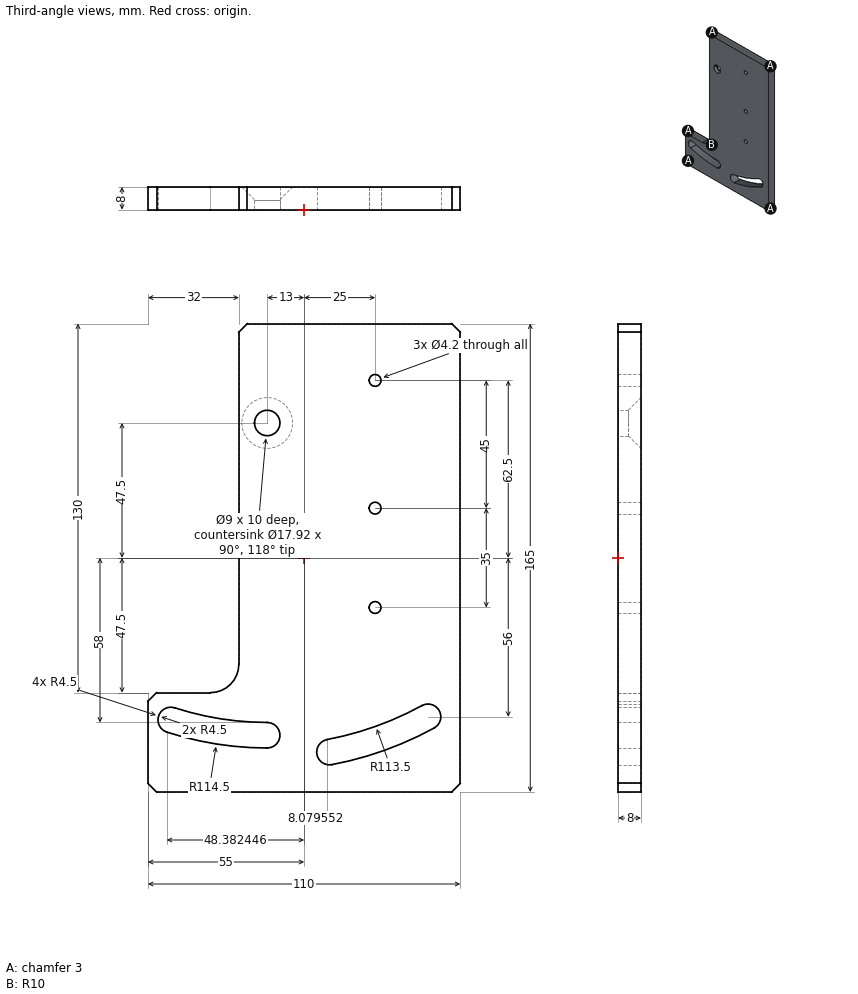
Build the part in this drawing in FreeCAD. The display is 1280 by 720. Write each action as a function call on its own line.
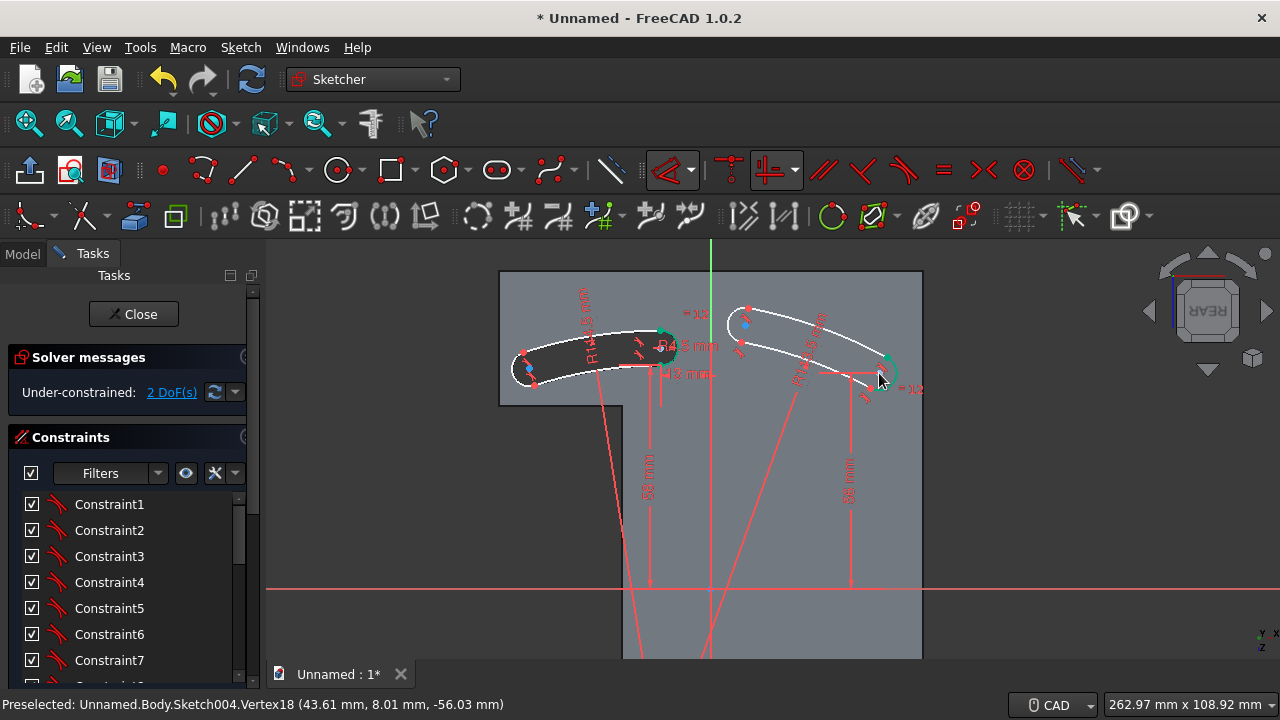
scroll(742, 342, up, 2)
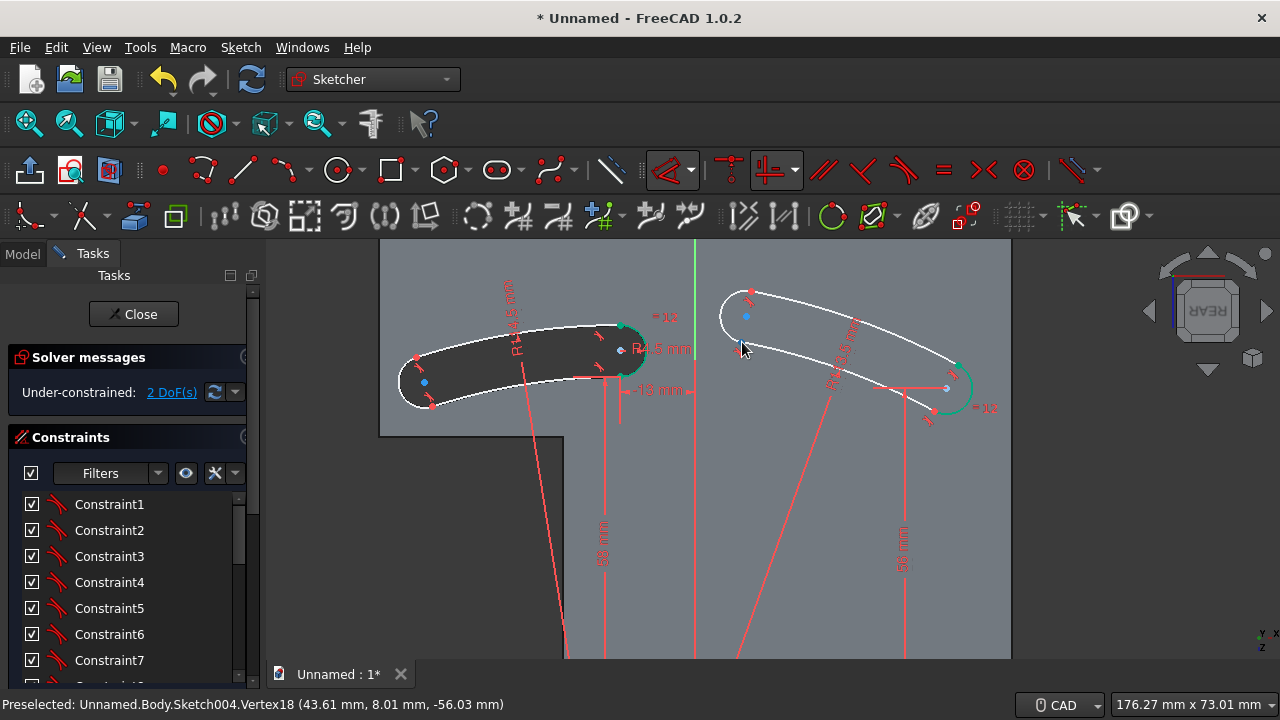
click(741, 342)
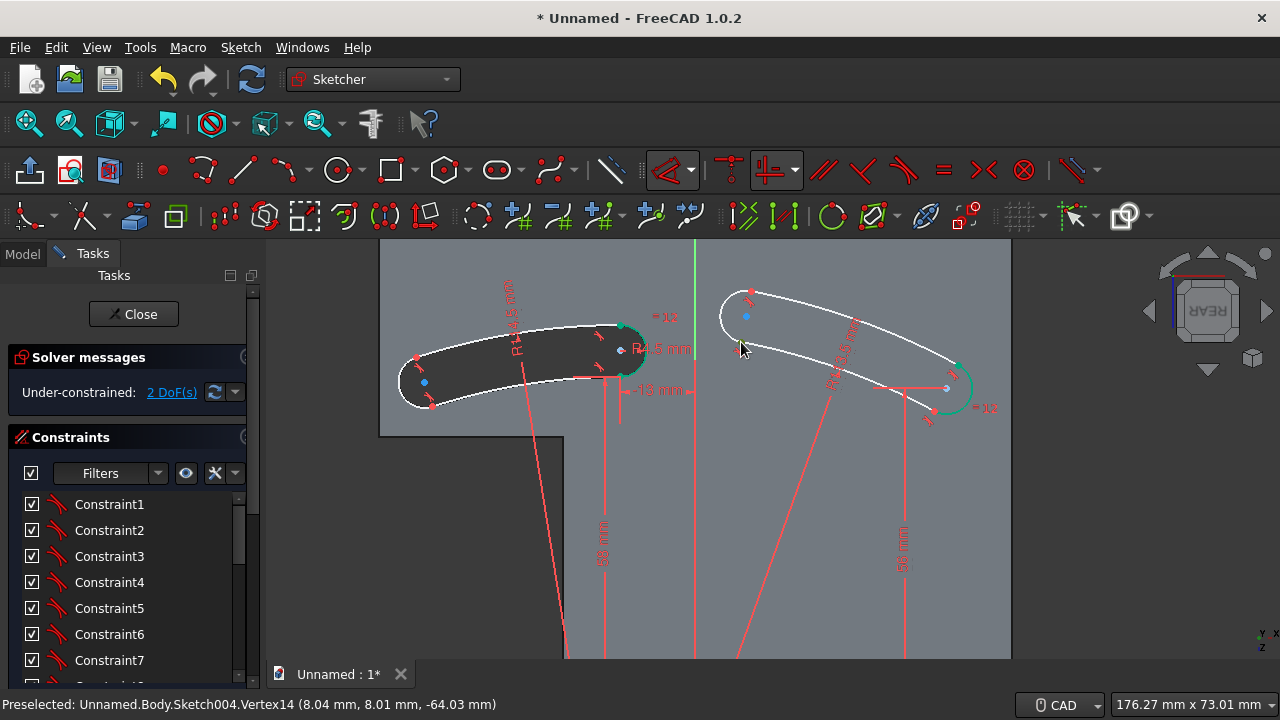
click(694, 170)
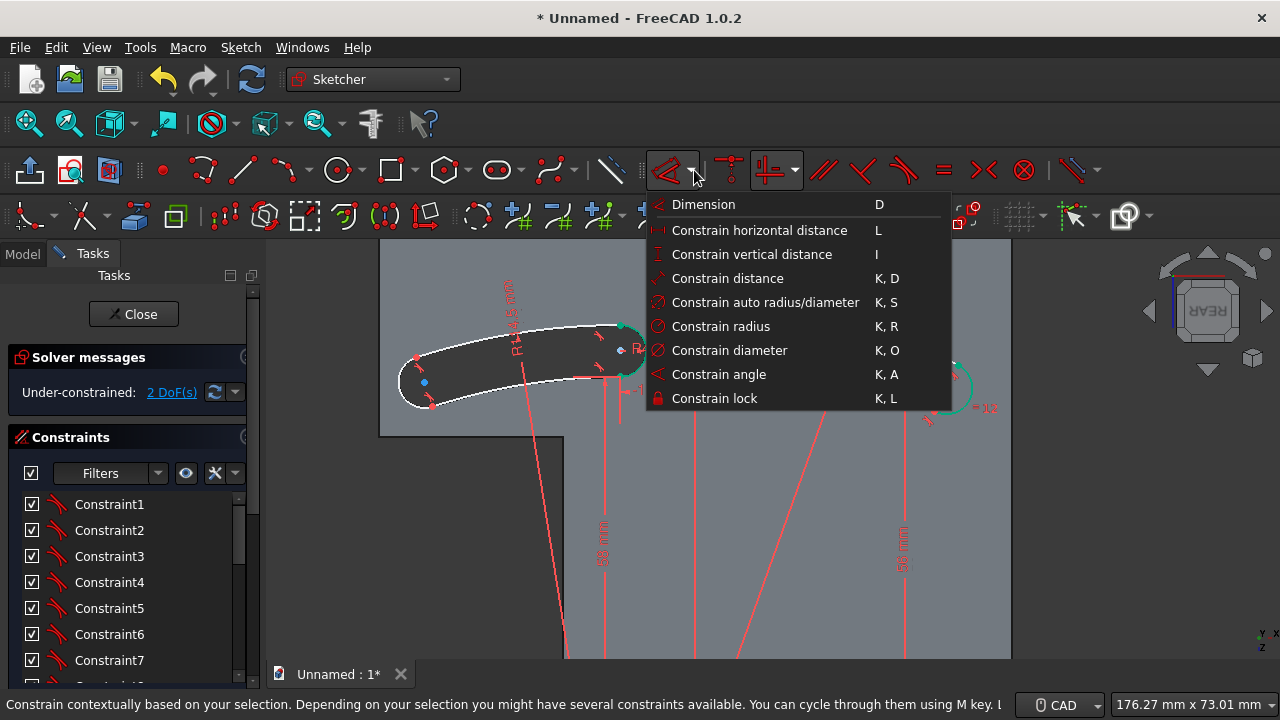
click(799, 230)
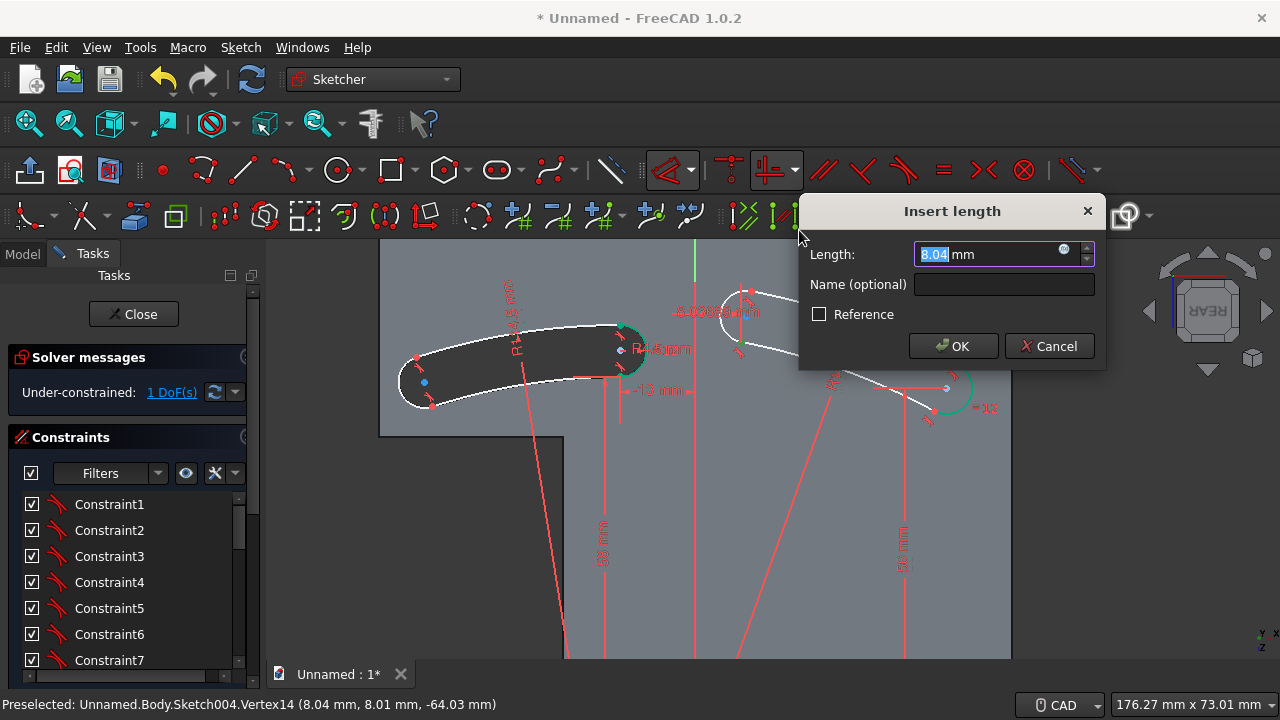
text(8.079552)
key(Return)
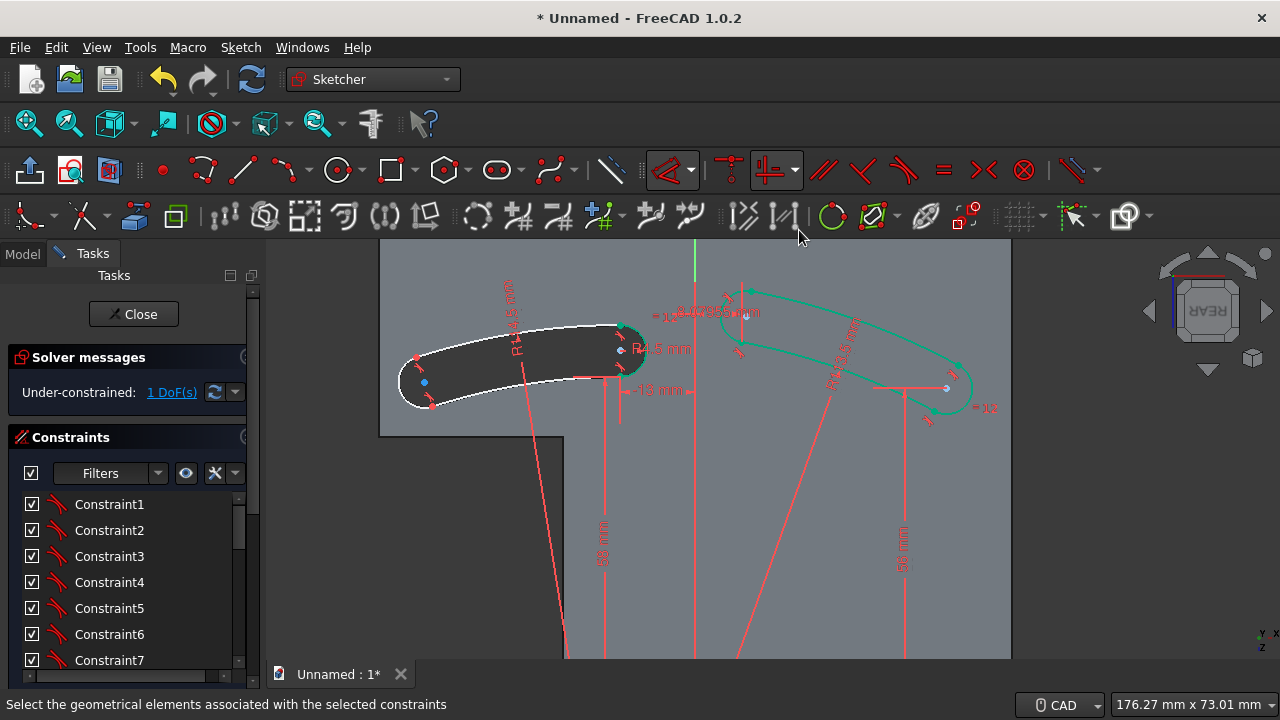
click(416, 357)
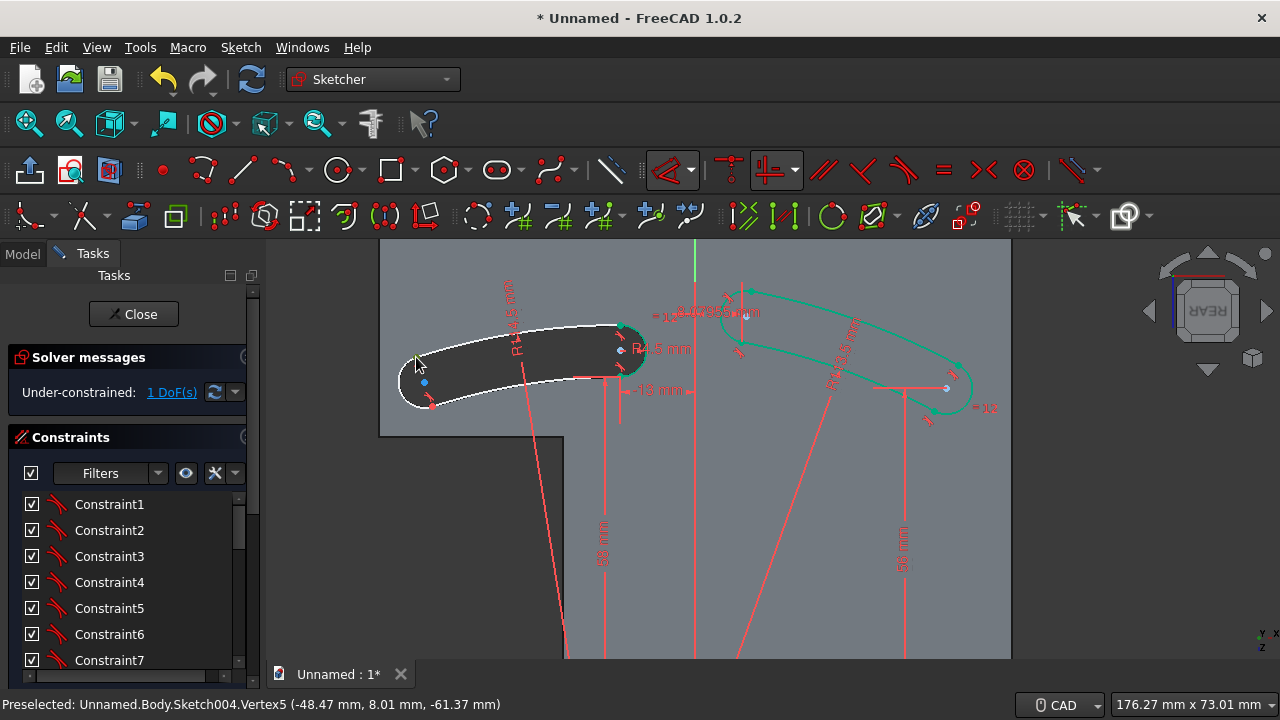
click(694, 170)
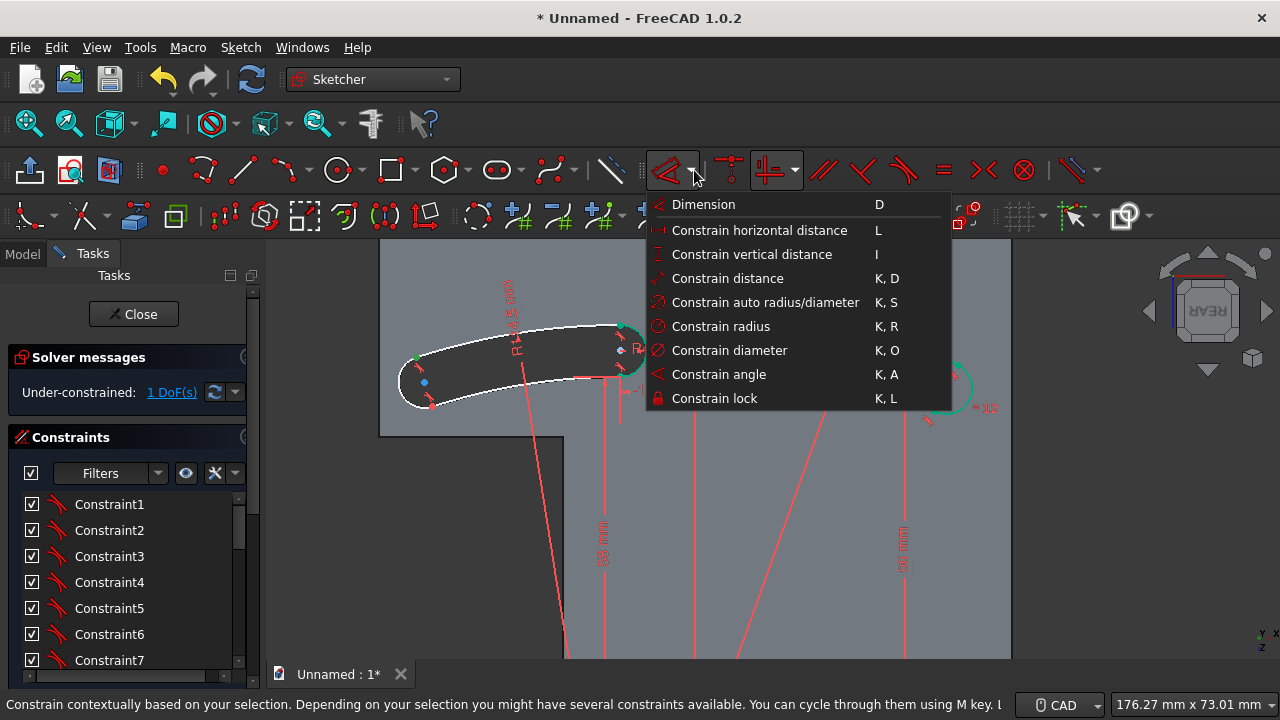
click(799, 230)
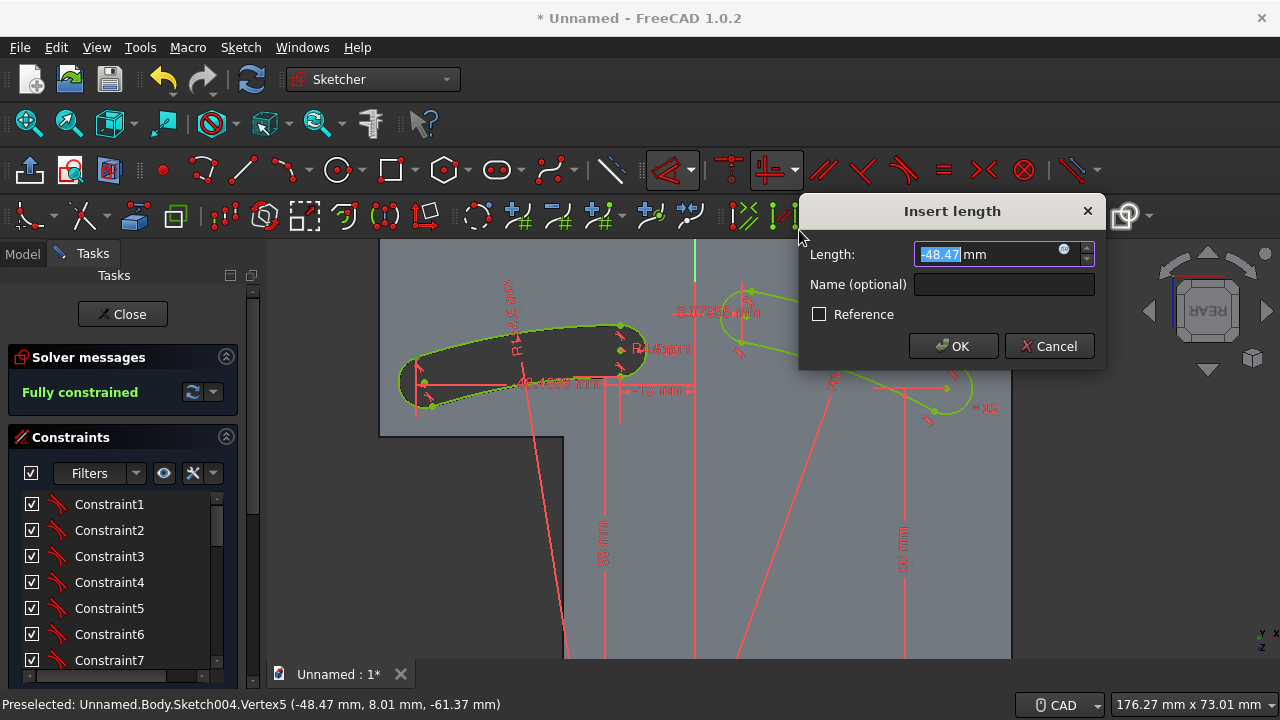
text(-48.382446)
key(Return)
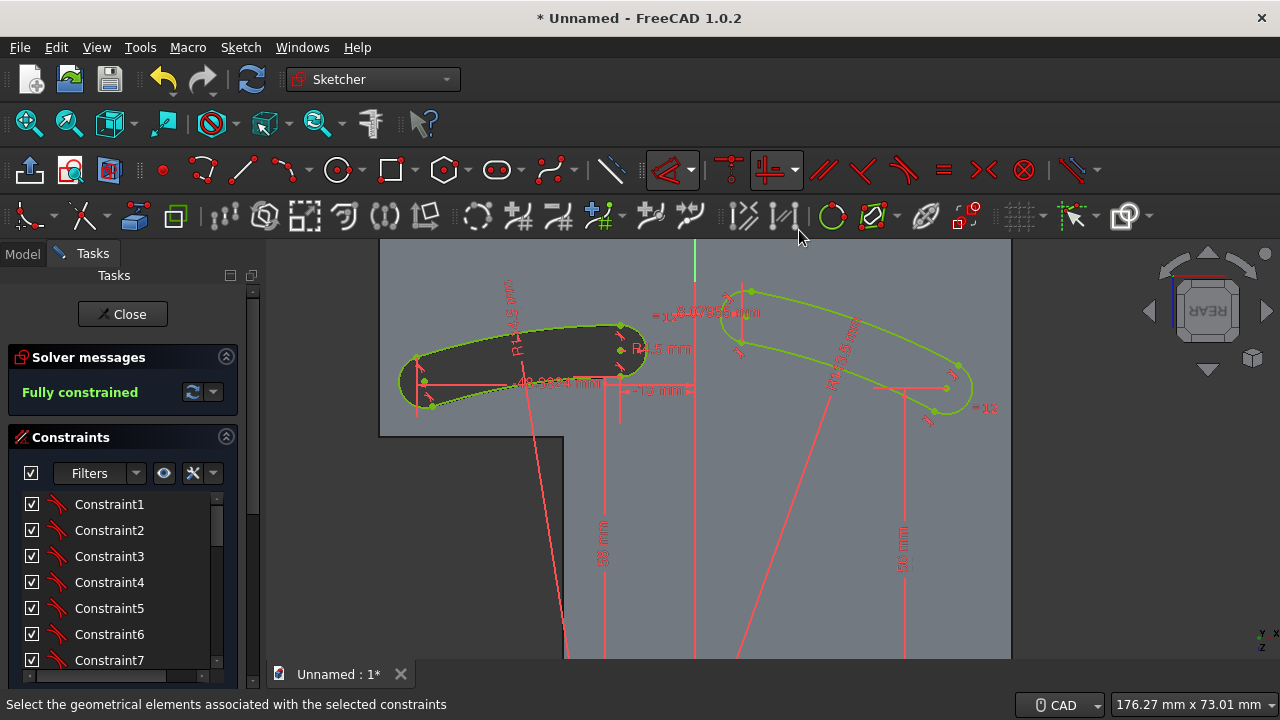
click(123, 314)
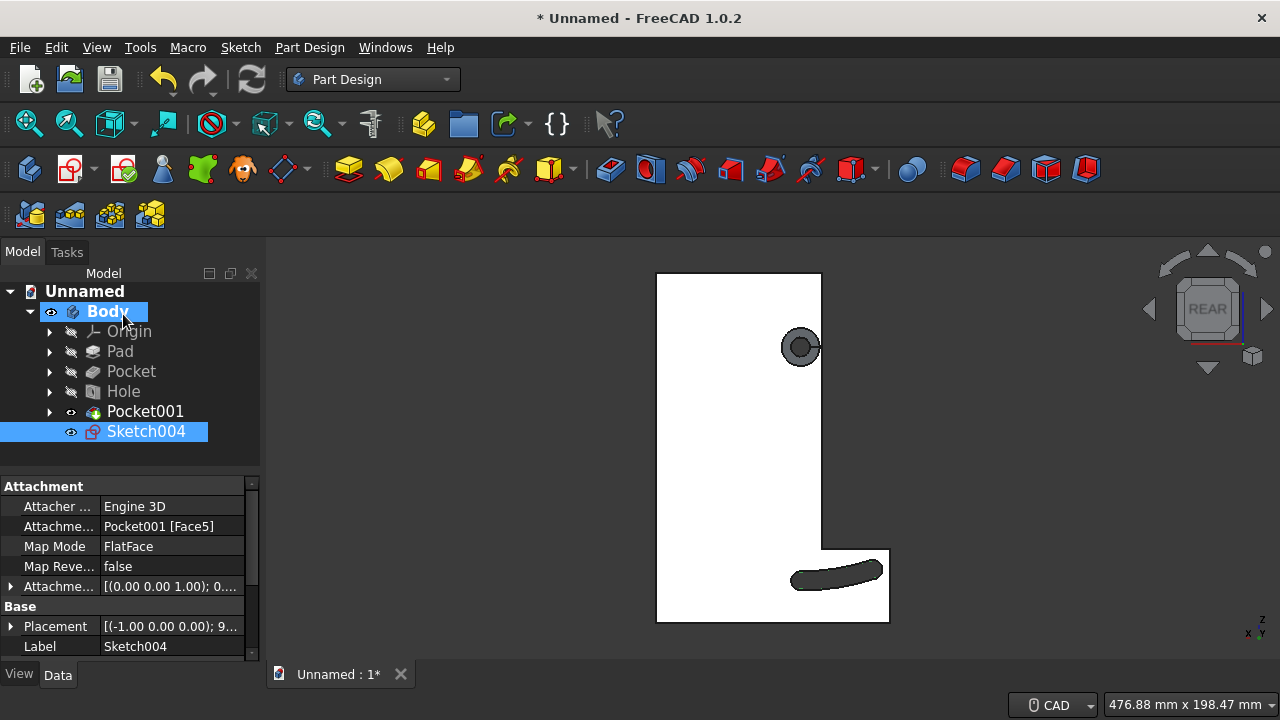
click(612, 170)